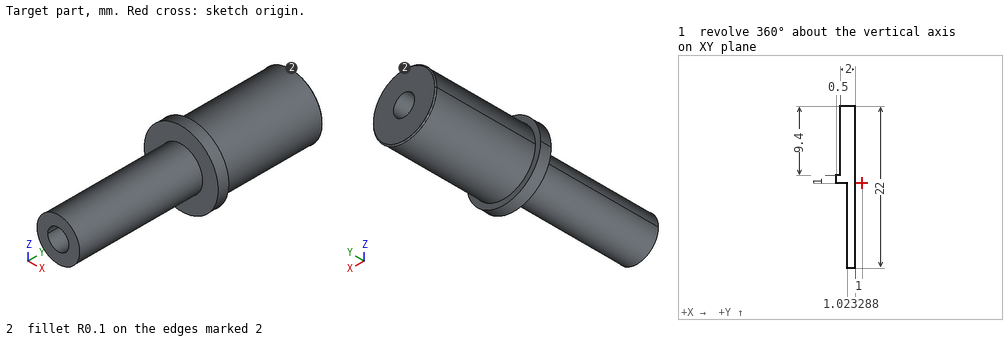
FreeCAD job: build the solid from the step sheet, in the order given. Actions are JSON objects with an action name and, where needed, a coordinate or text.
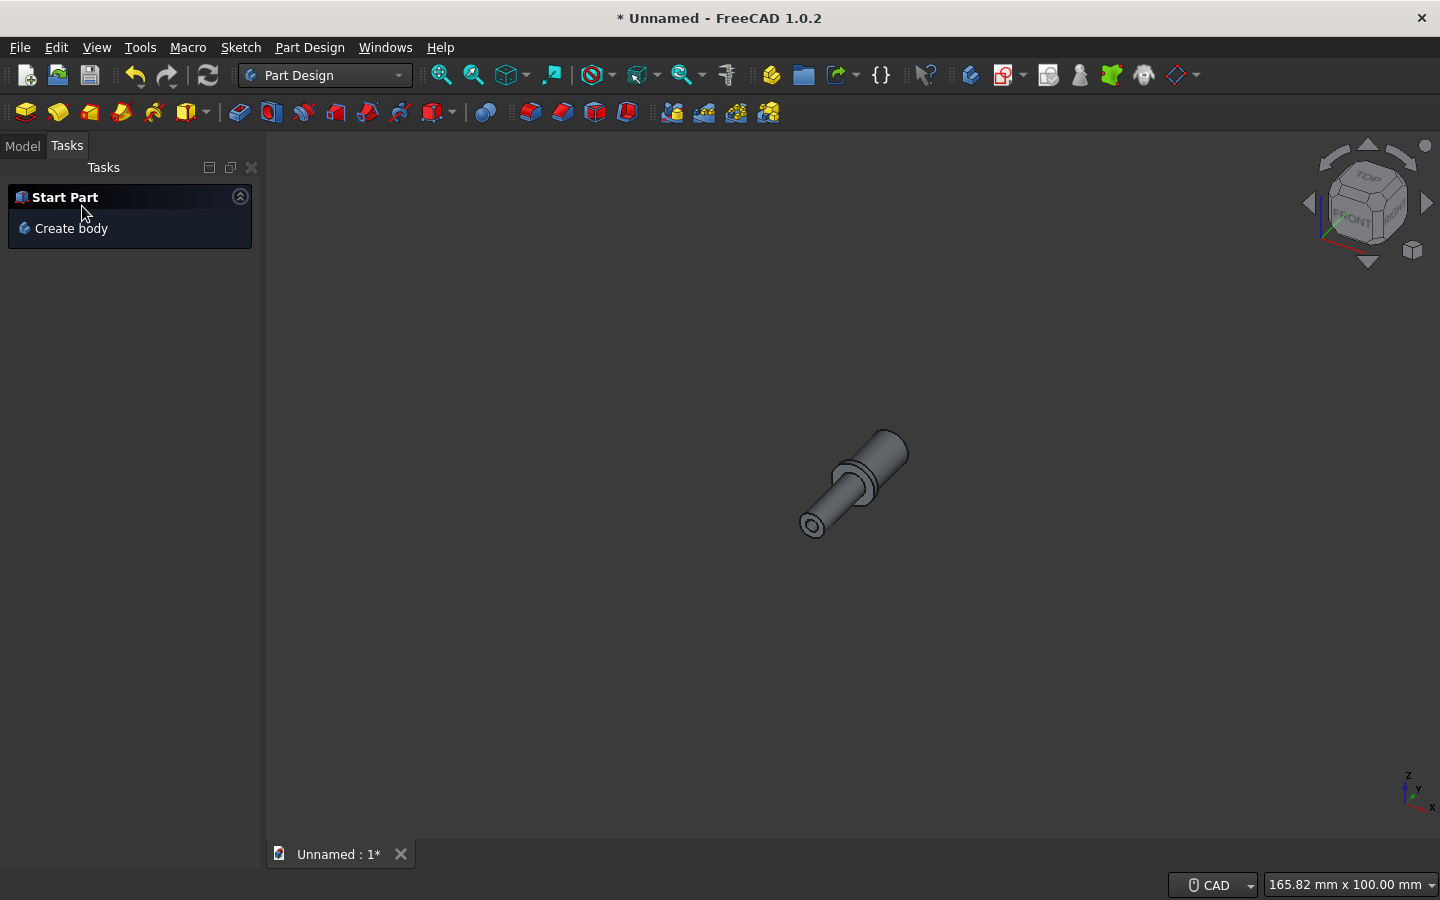
{"action": "left_click", "coordinate": [442, 76]}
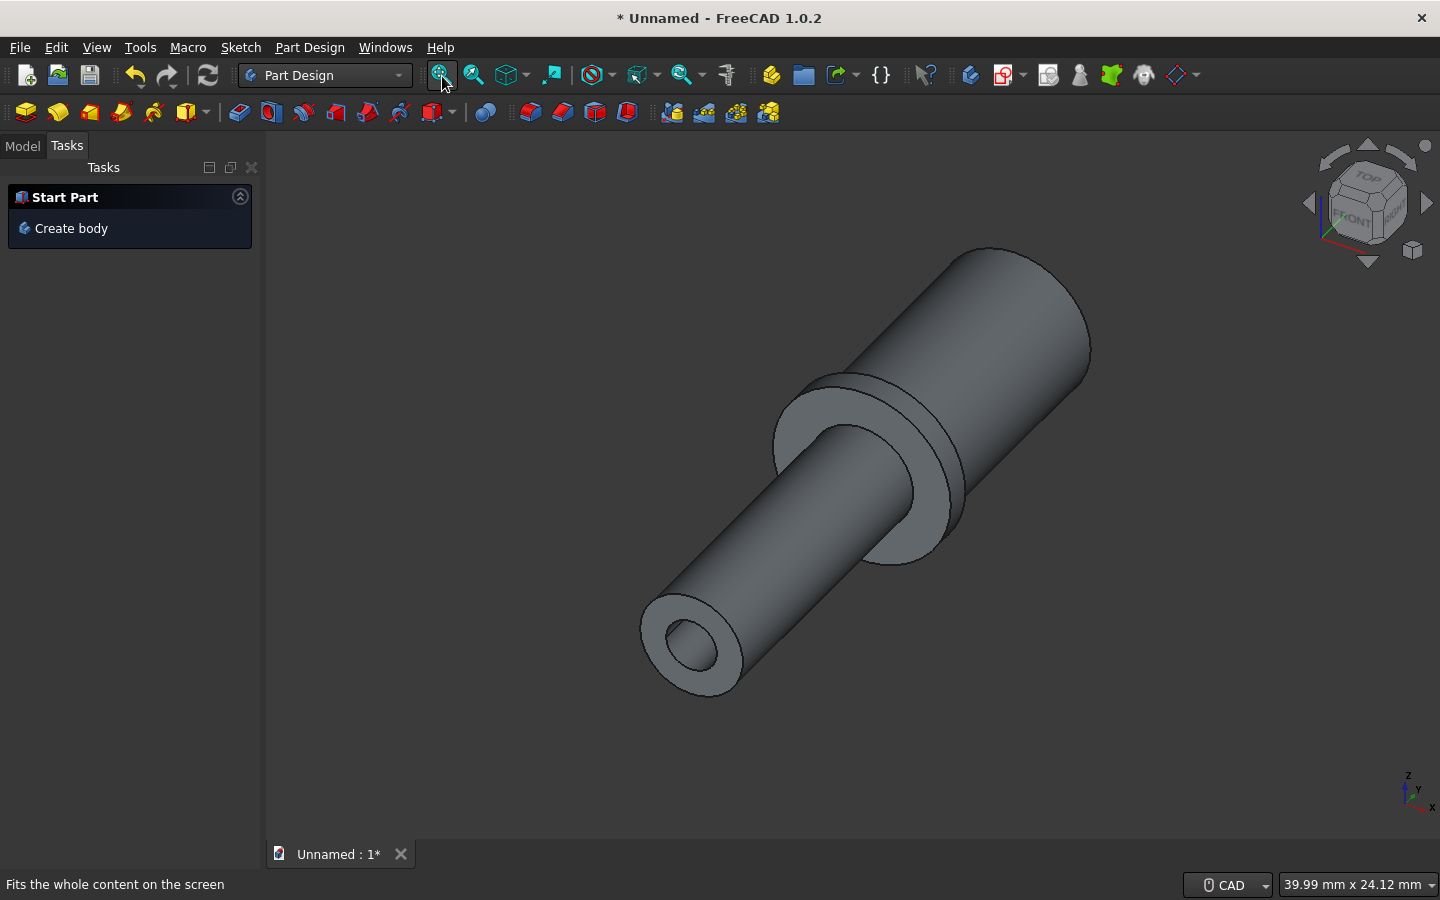
{"action": "key", "text": "0"}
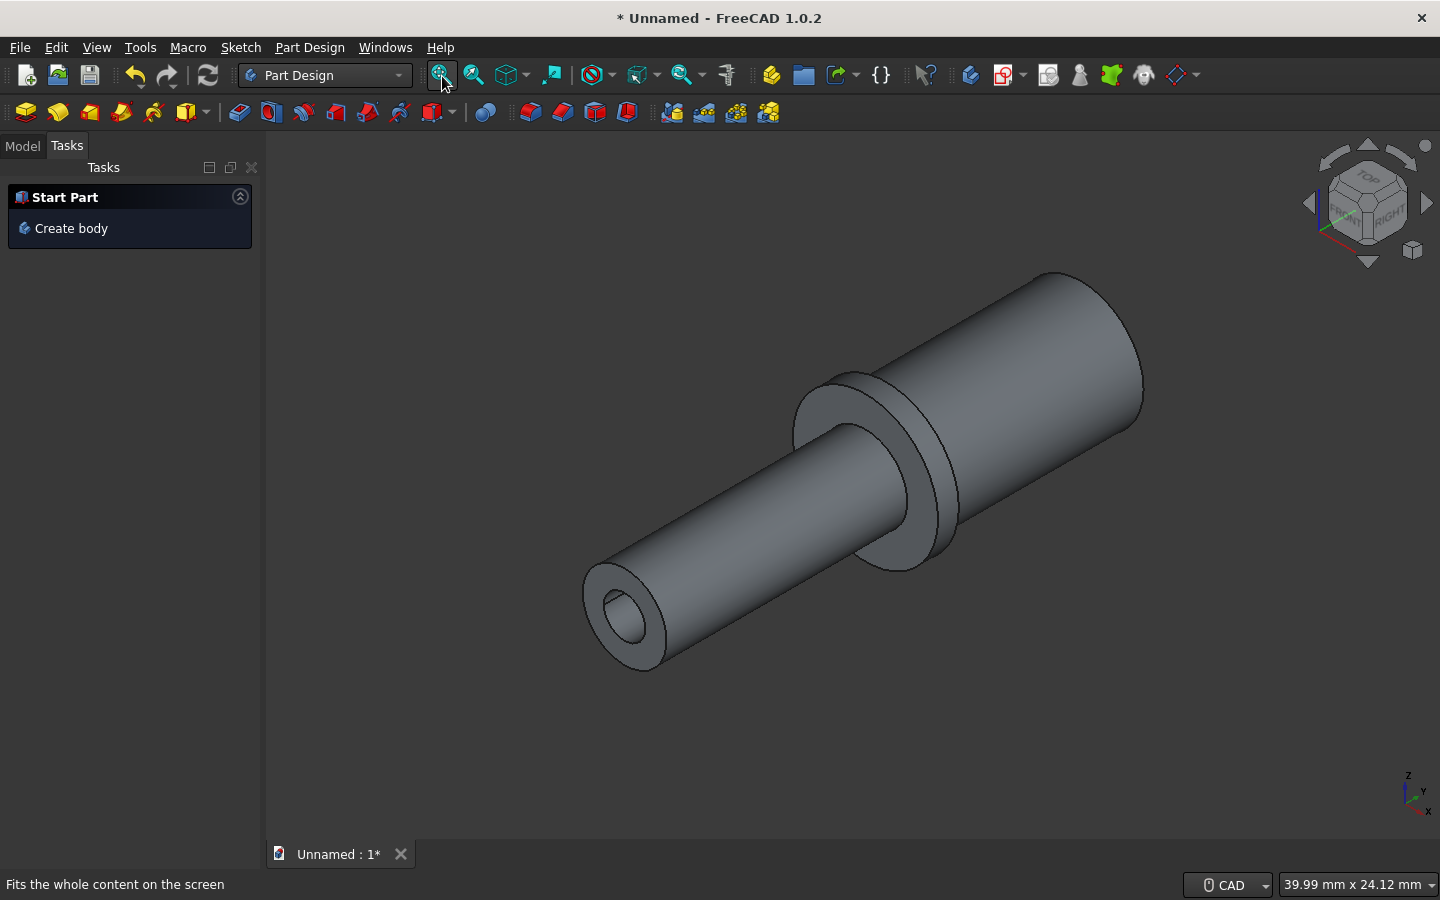
{"action": "left_click", "coordinate": [1101, 295]}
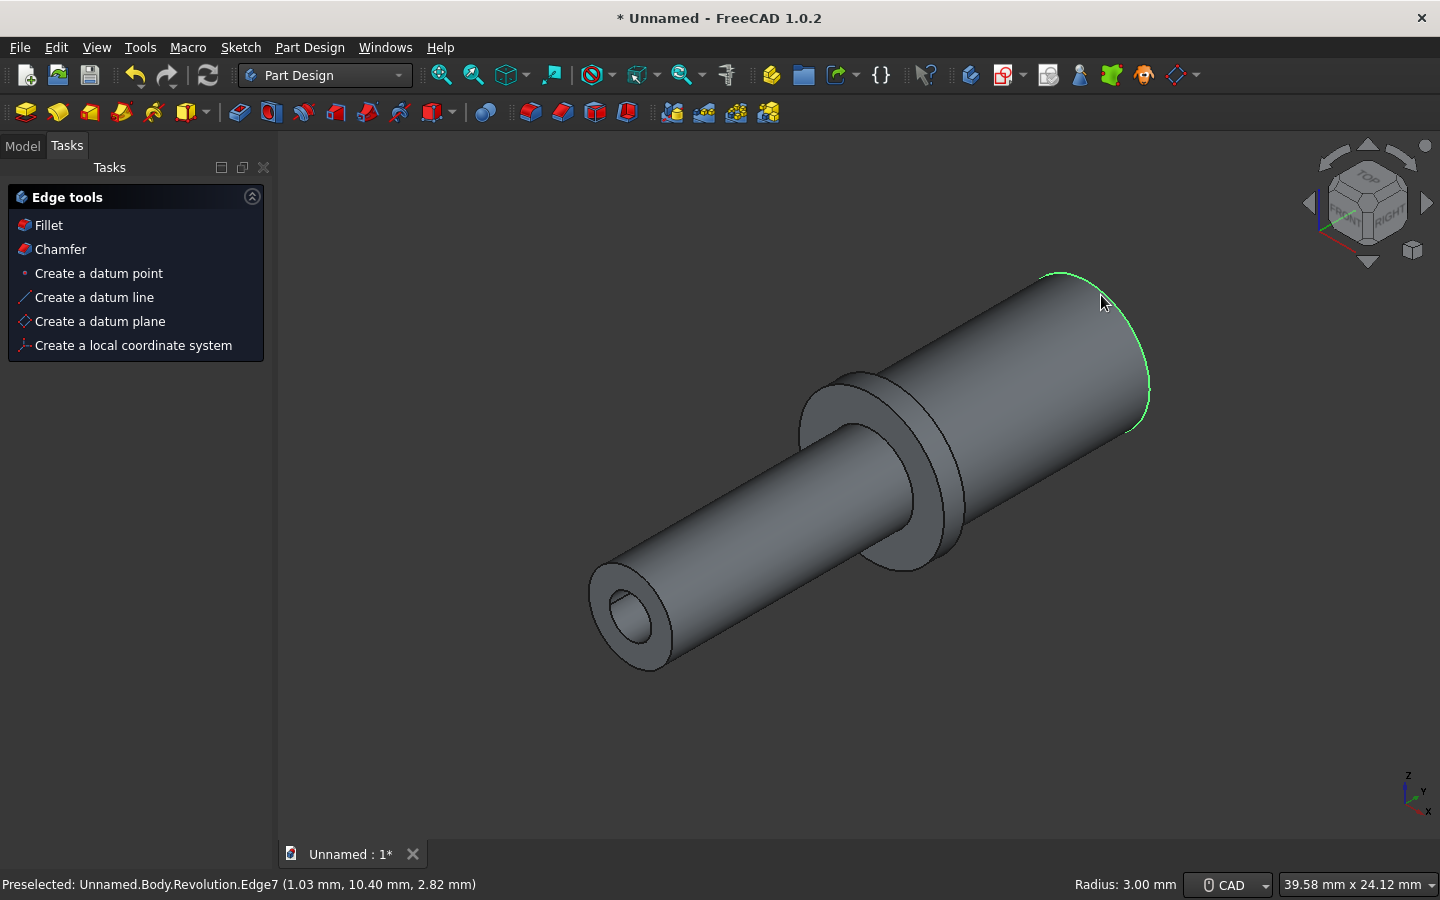
{"action": "left_click", "coordinate": [532, 112]}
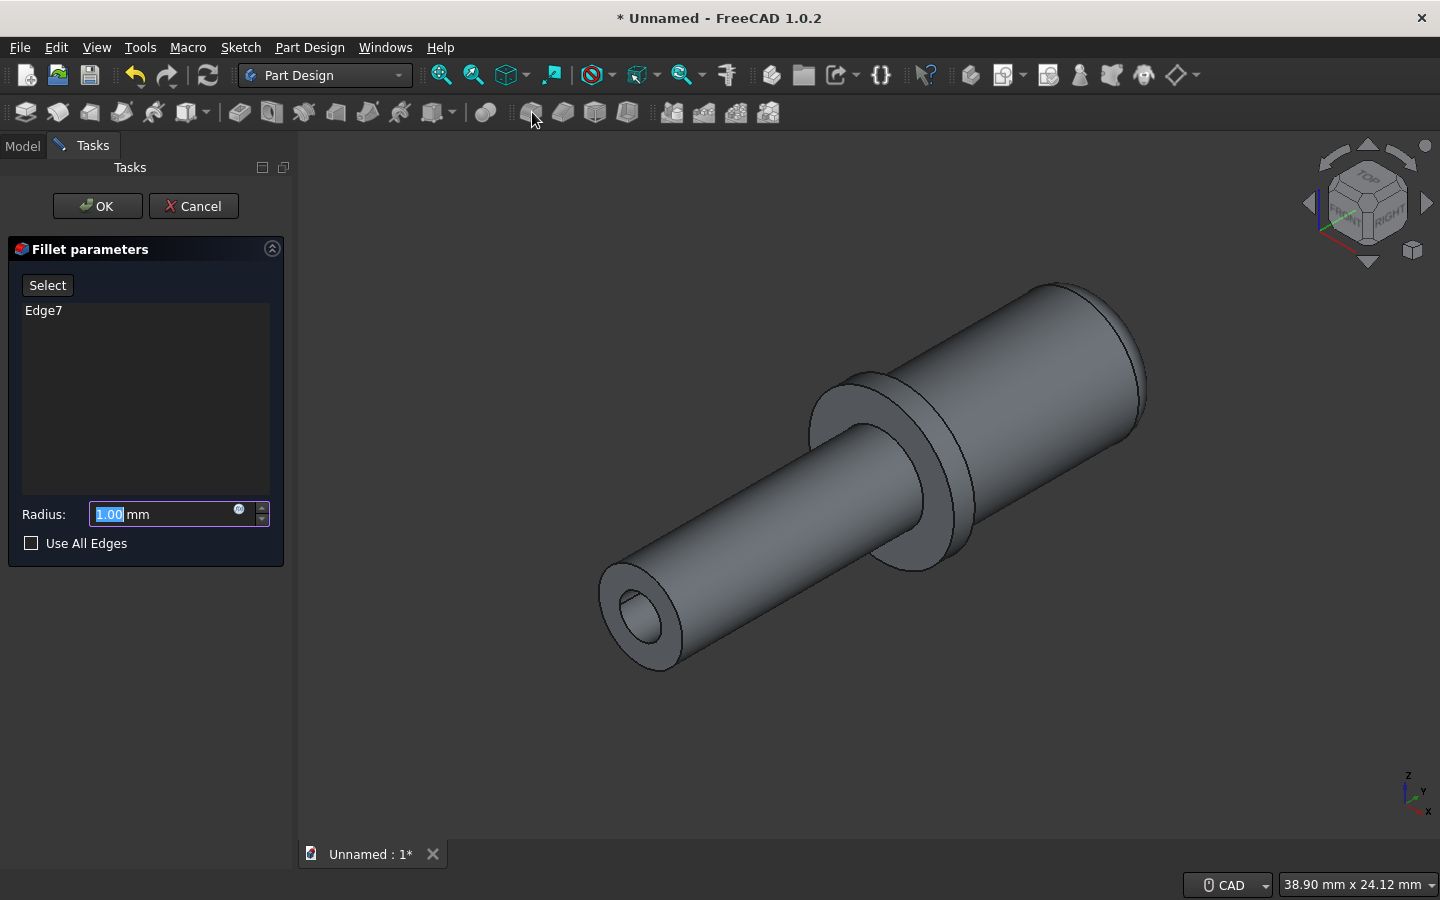
{"action": "type", "text": "0.1"}
{"action": "key", "text": "Tab"}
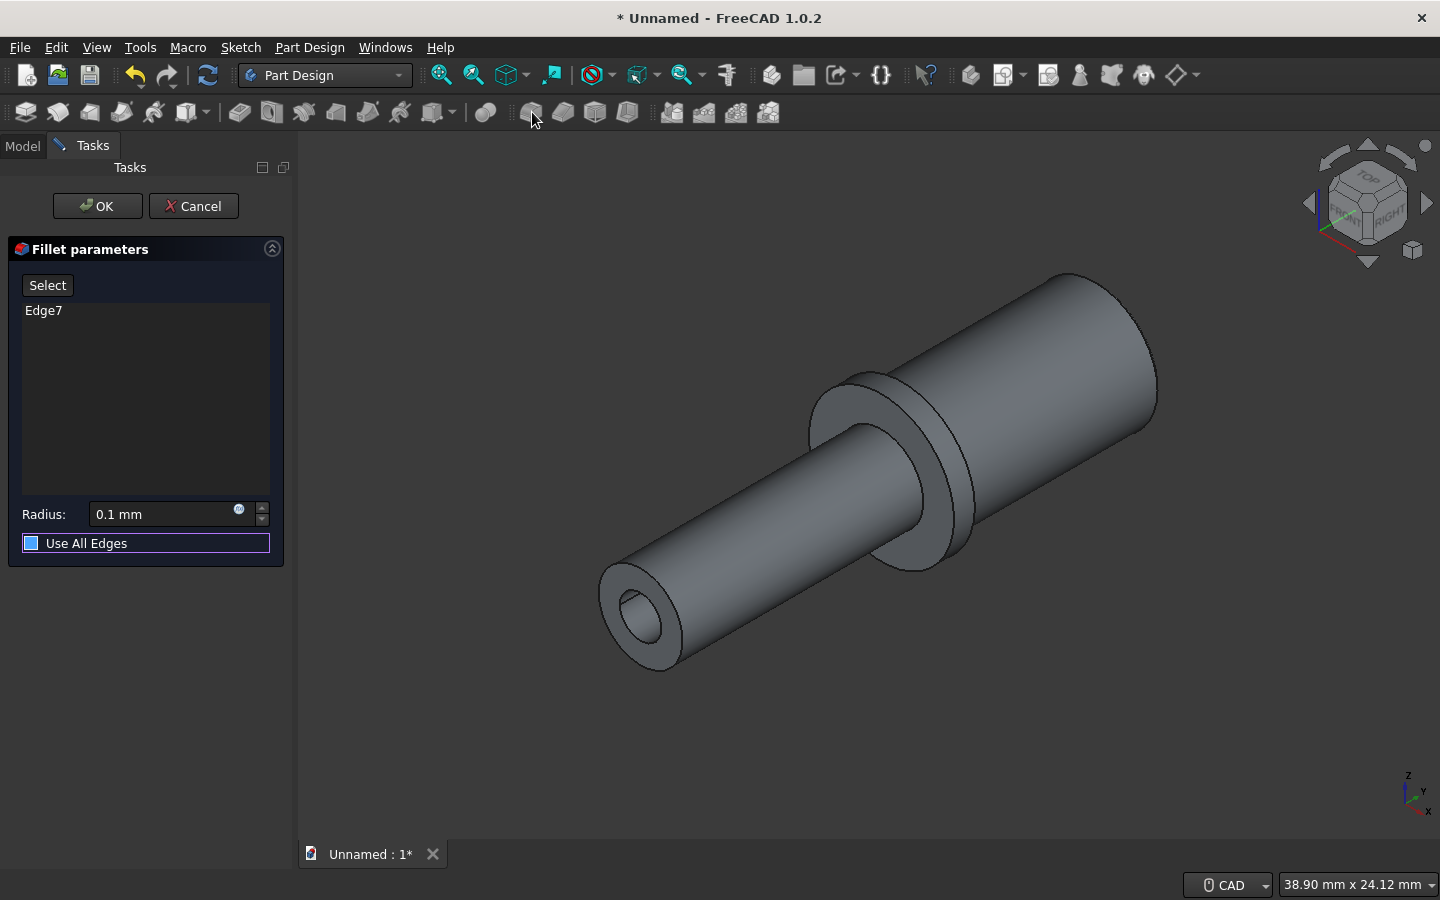
{"action": "left_click", "coordinate": [98, 206]}